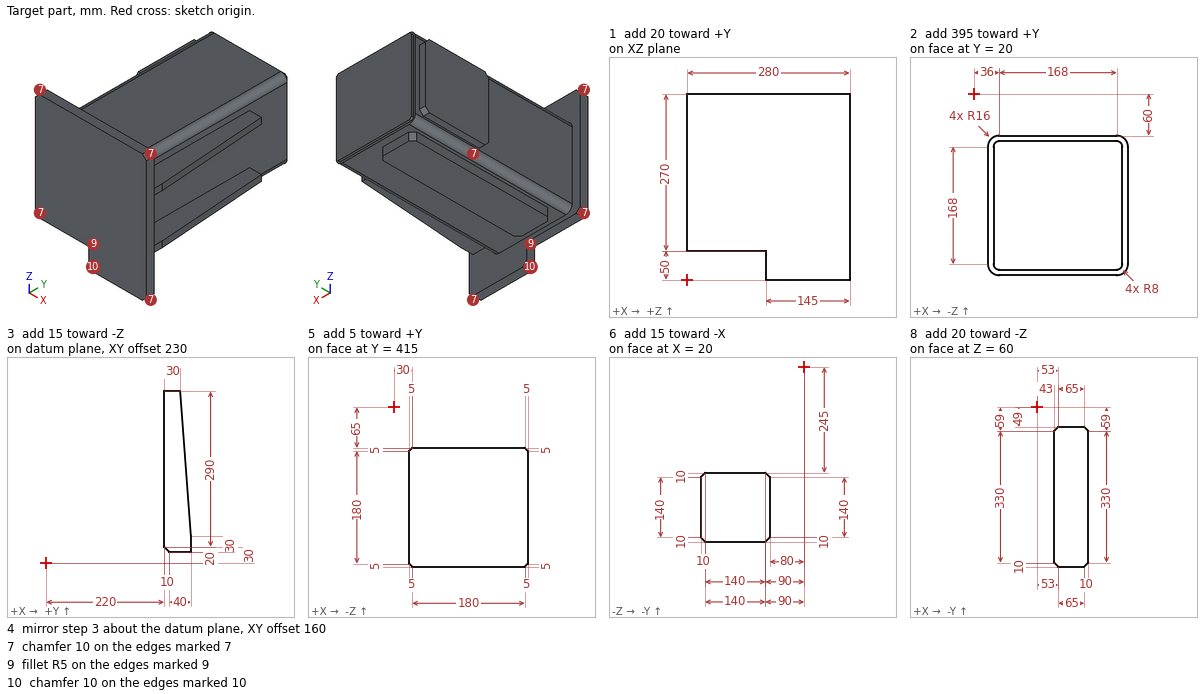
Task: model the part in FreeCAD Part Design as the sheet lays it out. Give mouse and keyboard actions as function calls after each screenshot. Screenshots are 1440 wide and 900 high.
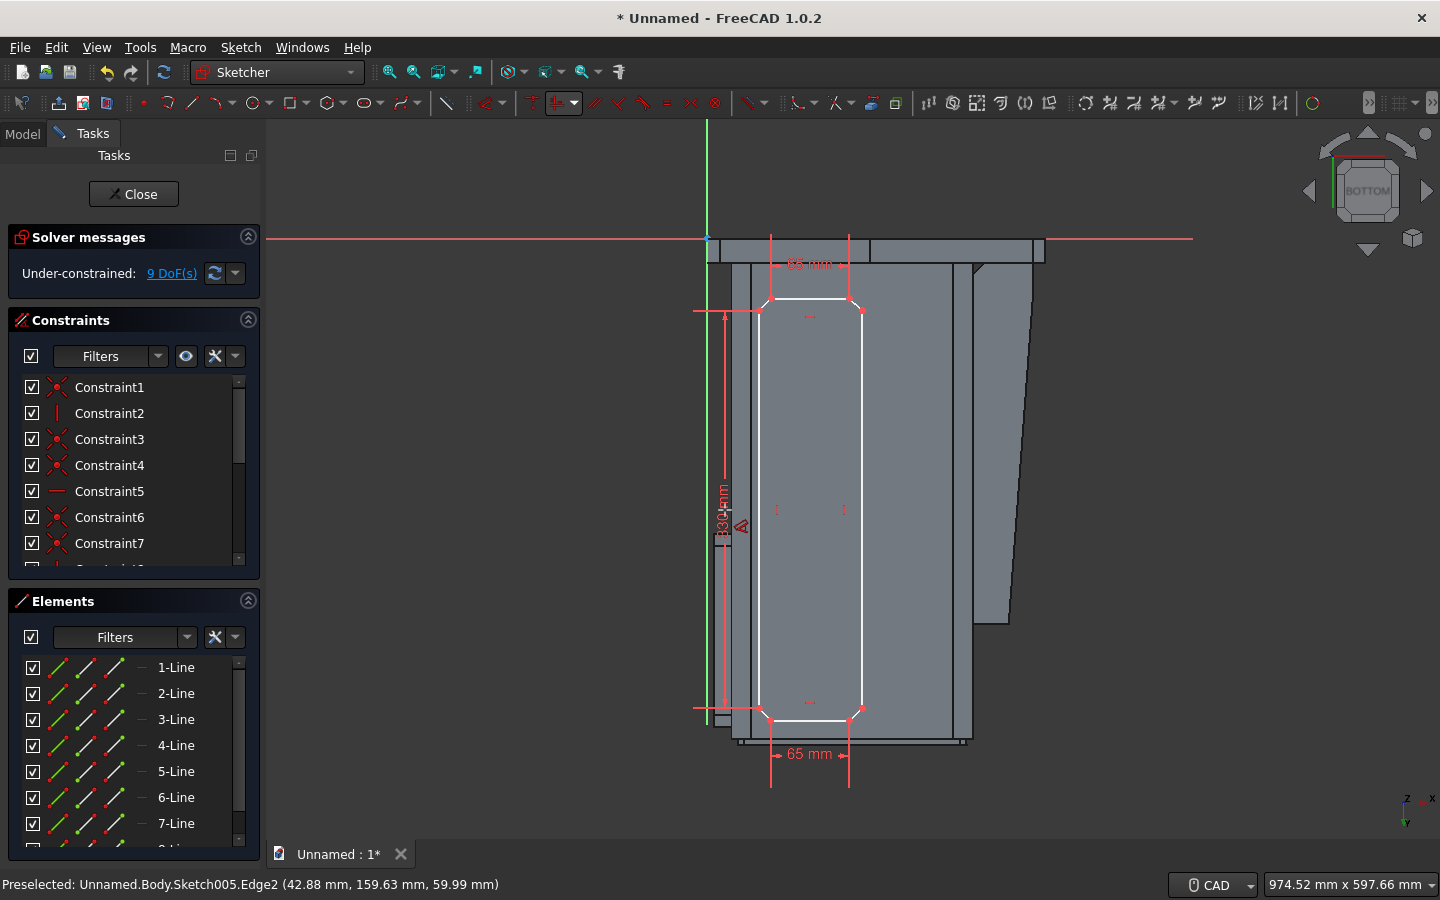
click(862, 589)
click(896, 510)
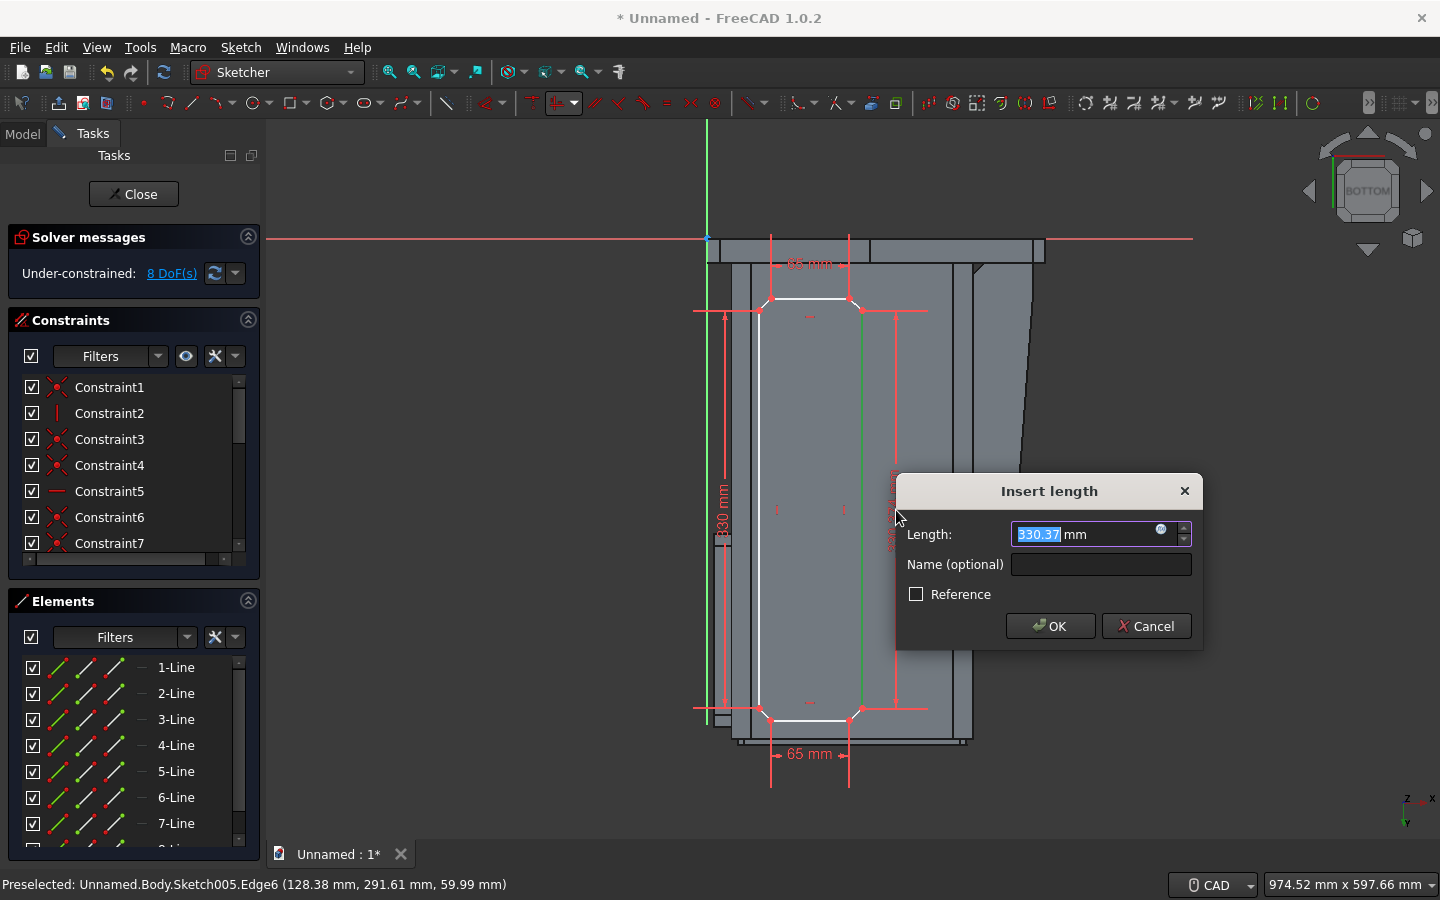
text(330)
key(Return)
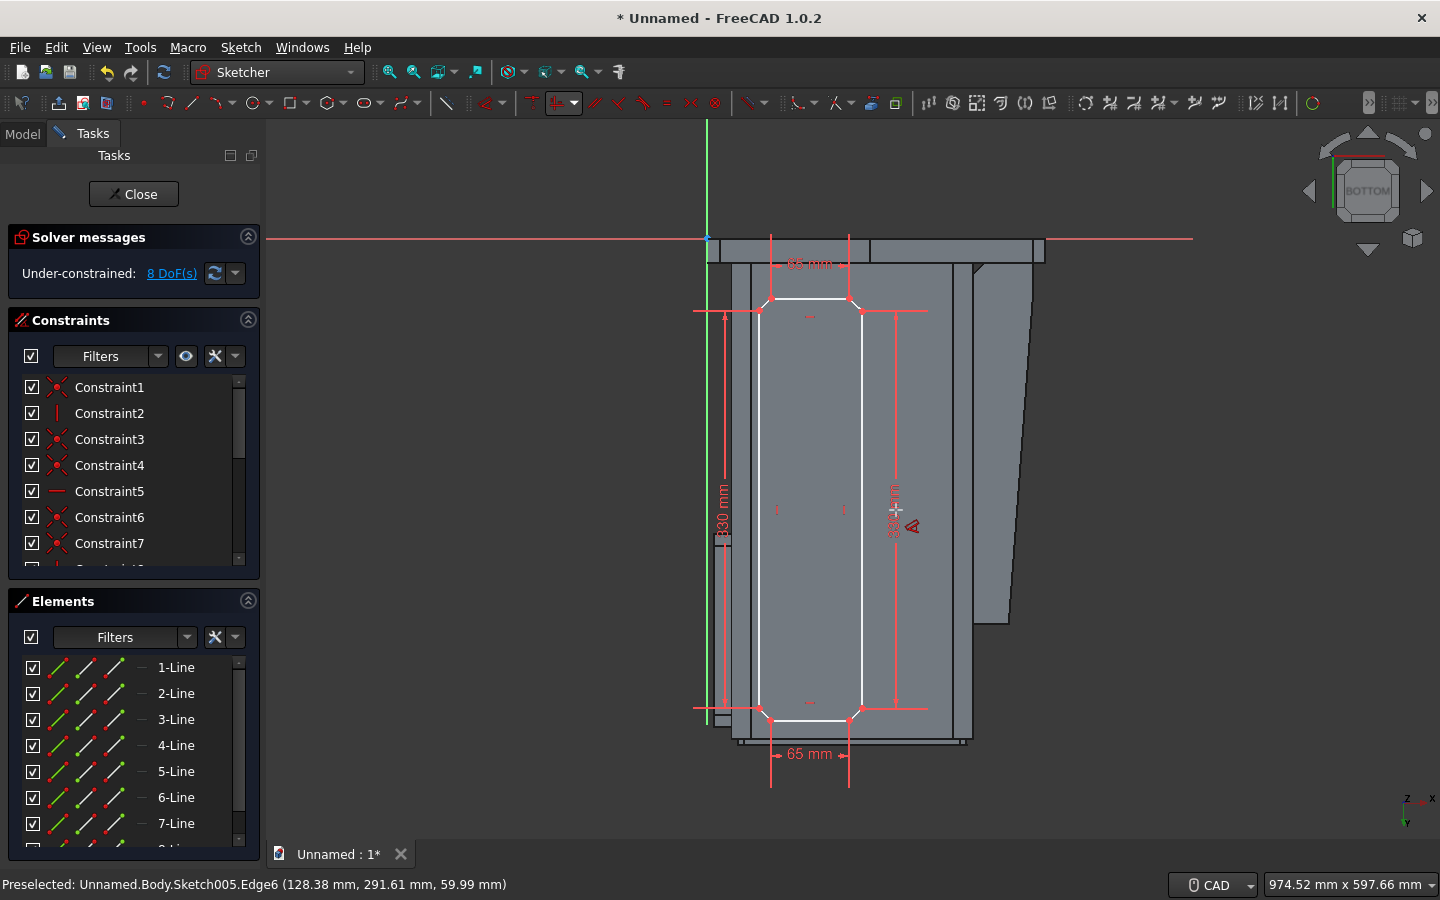
click(771, 299)
click(739, 205)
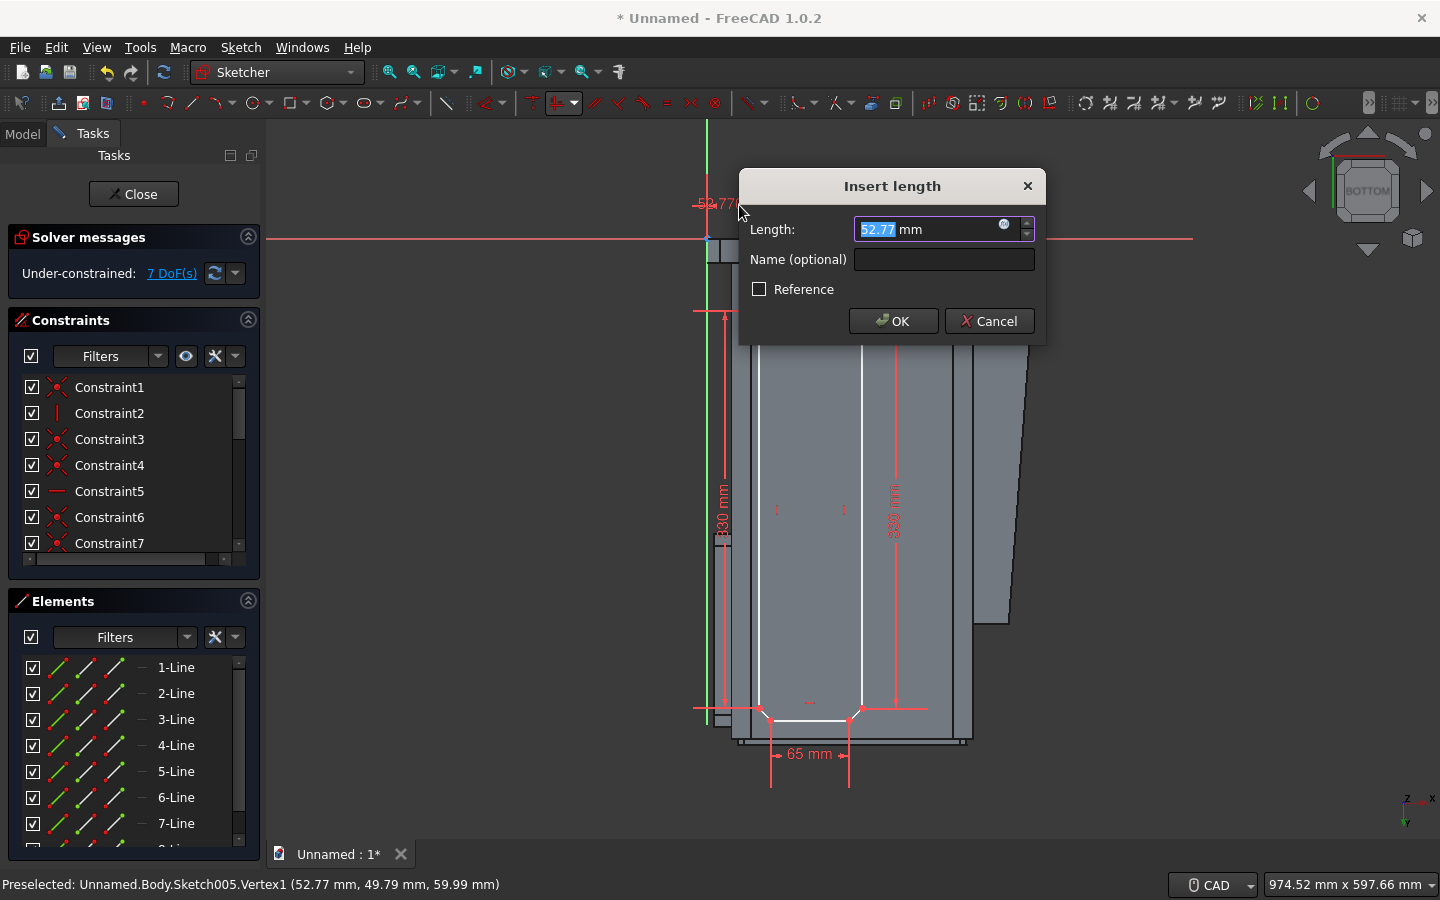
text(53)
key(Return)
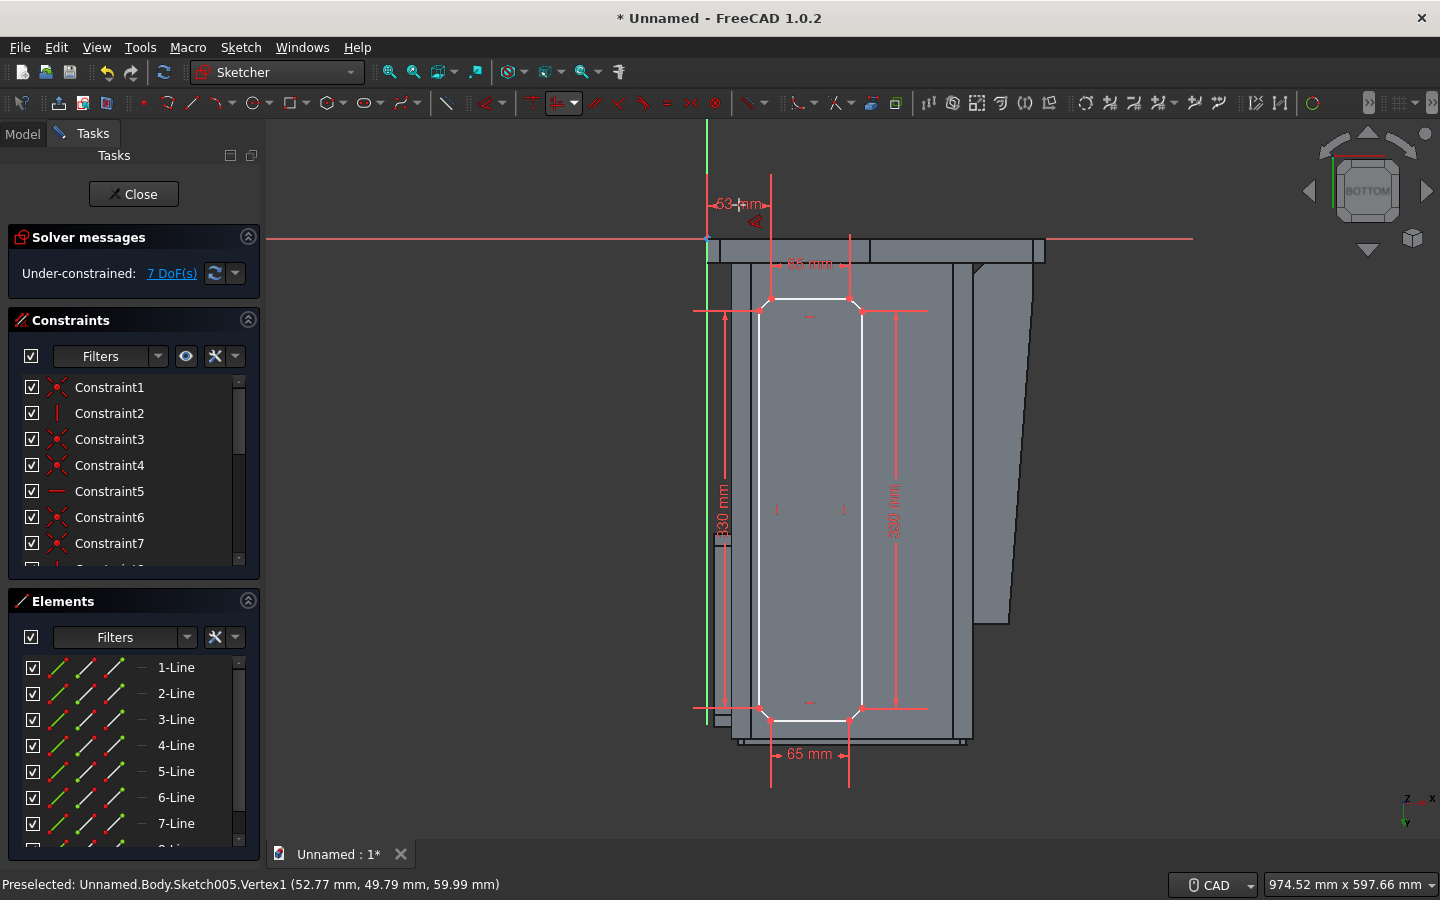
click(771, 299)
click(673, 269)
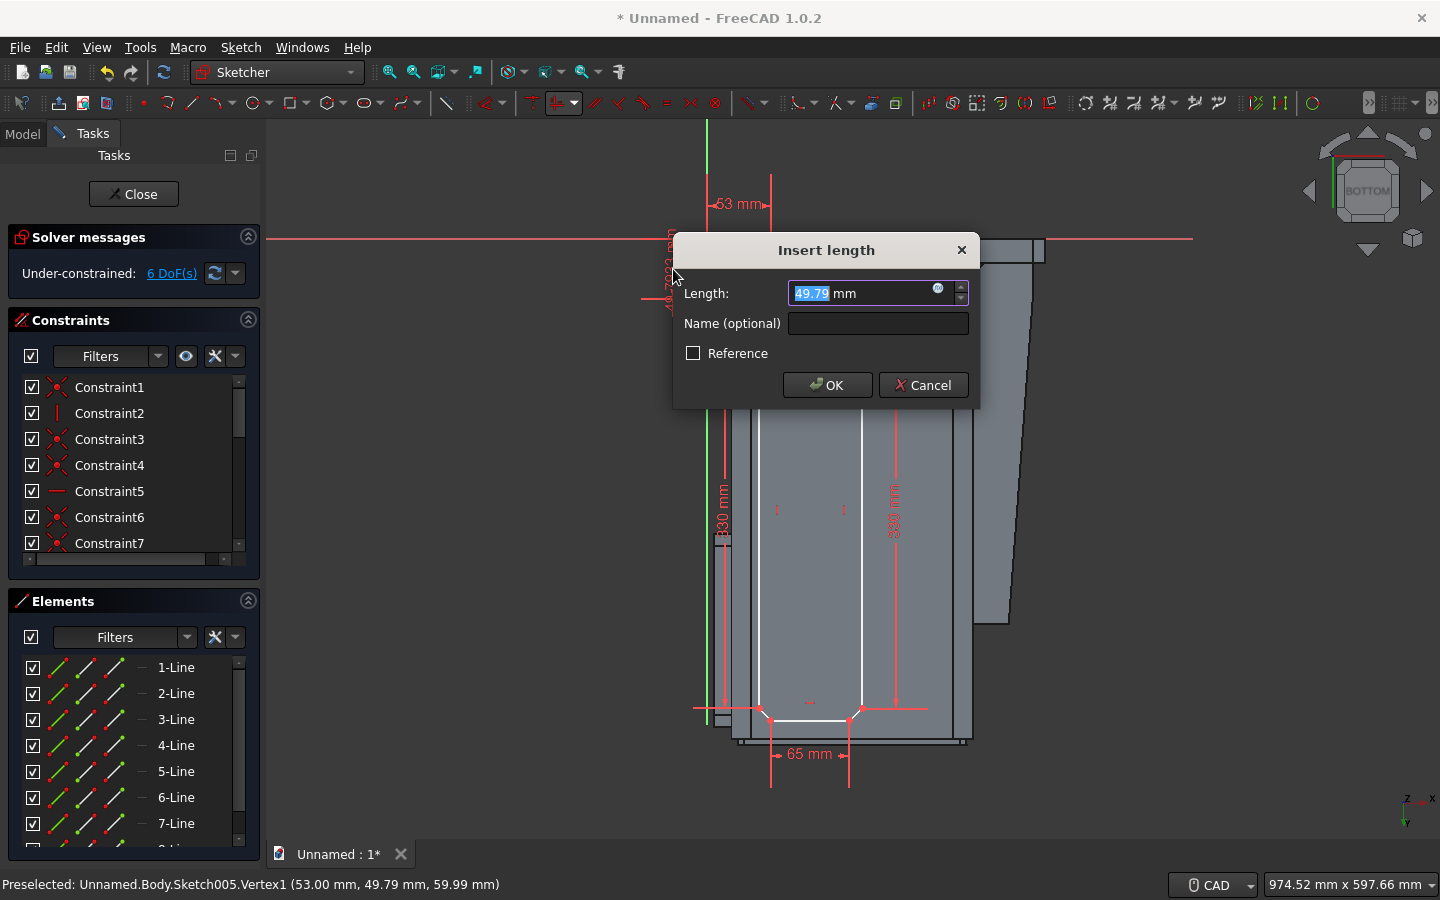
text(49)
key(Return)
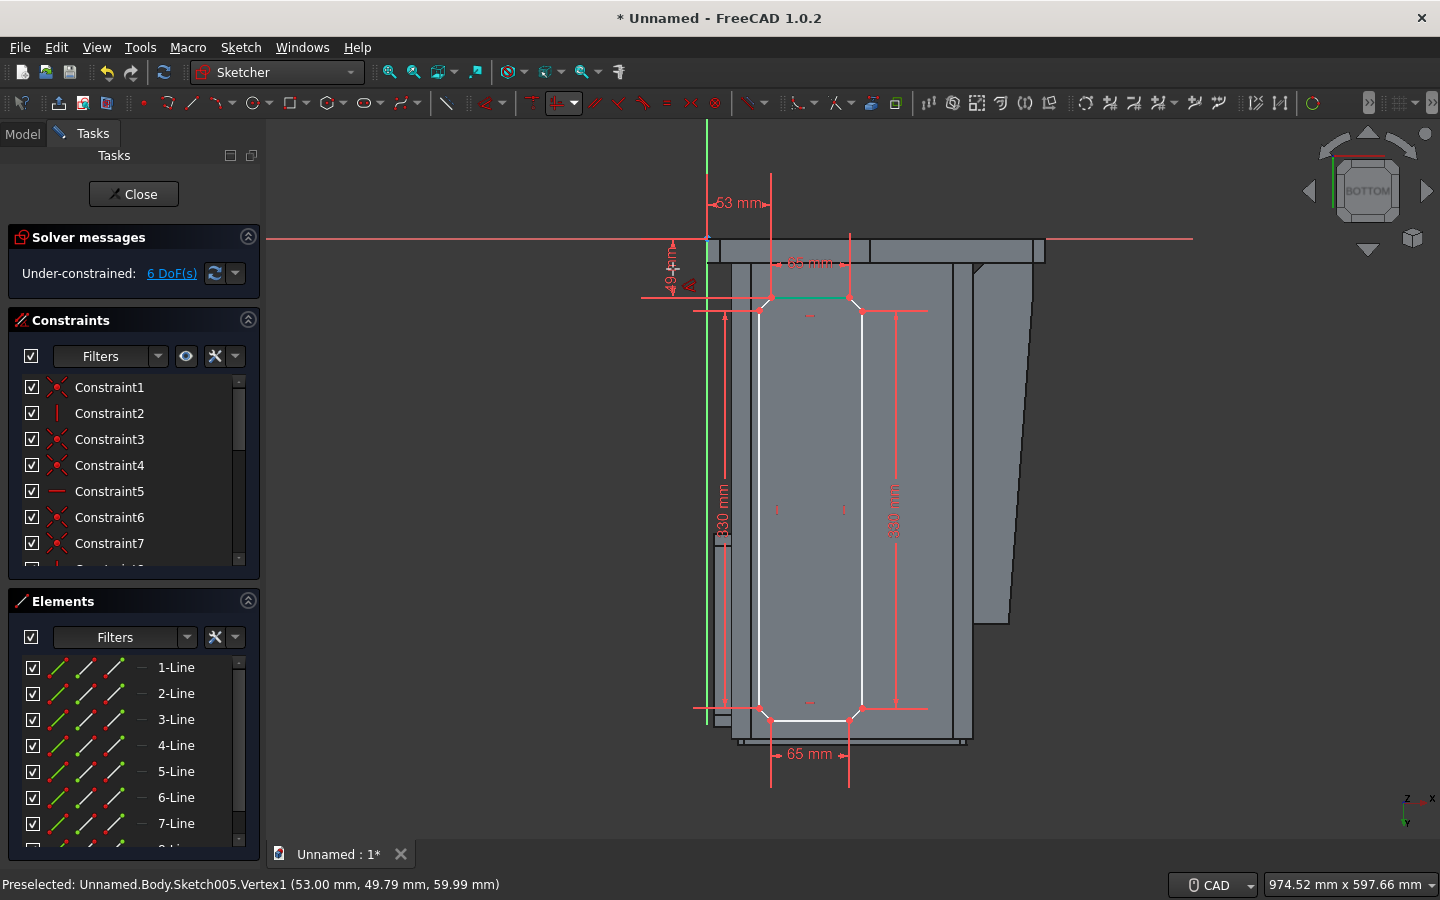
click(759, 311)
click(733, 345)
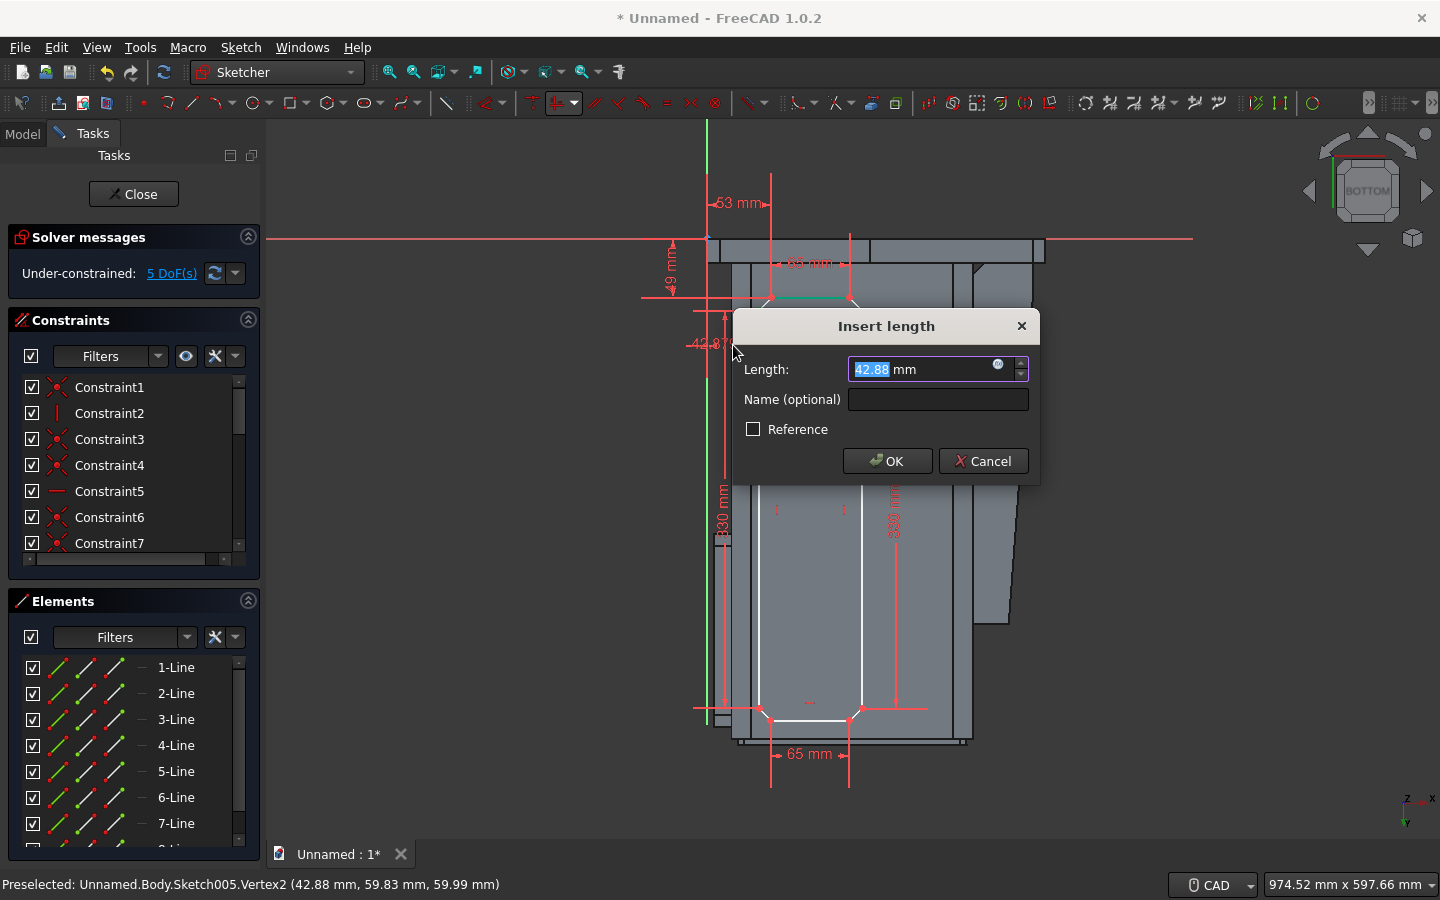
text(43)
key(Return)